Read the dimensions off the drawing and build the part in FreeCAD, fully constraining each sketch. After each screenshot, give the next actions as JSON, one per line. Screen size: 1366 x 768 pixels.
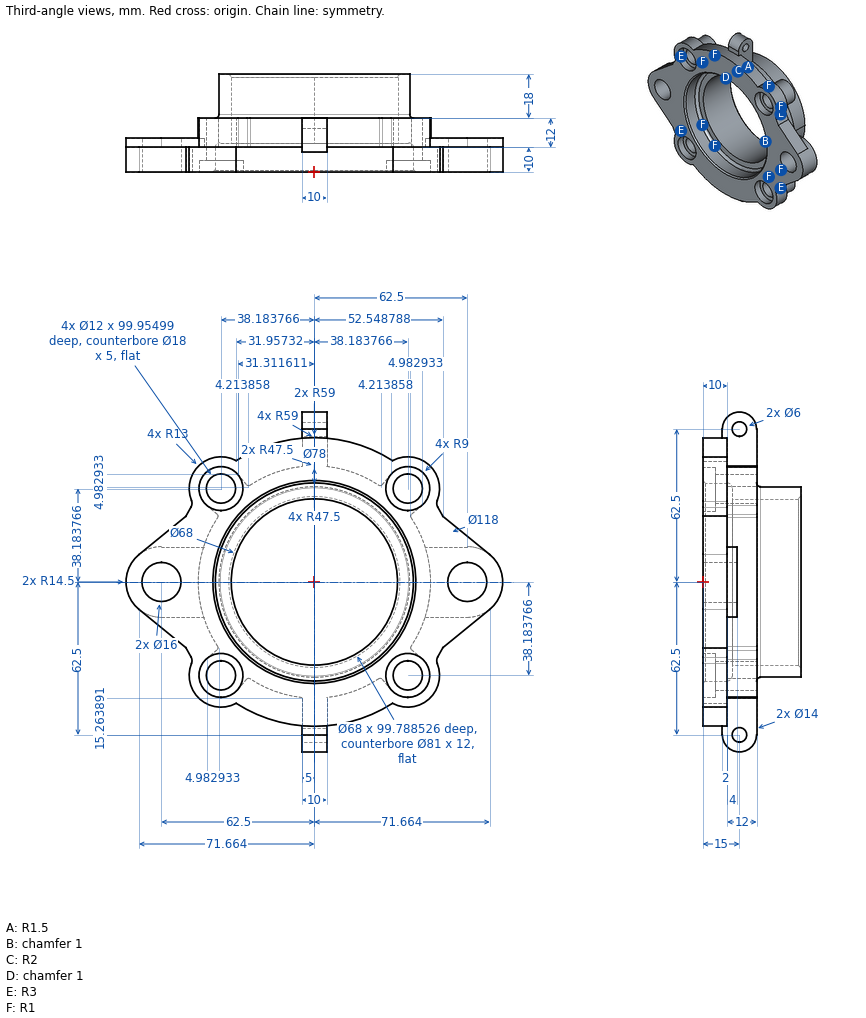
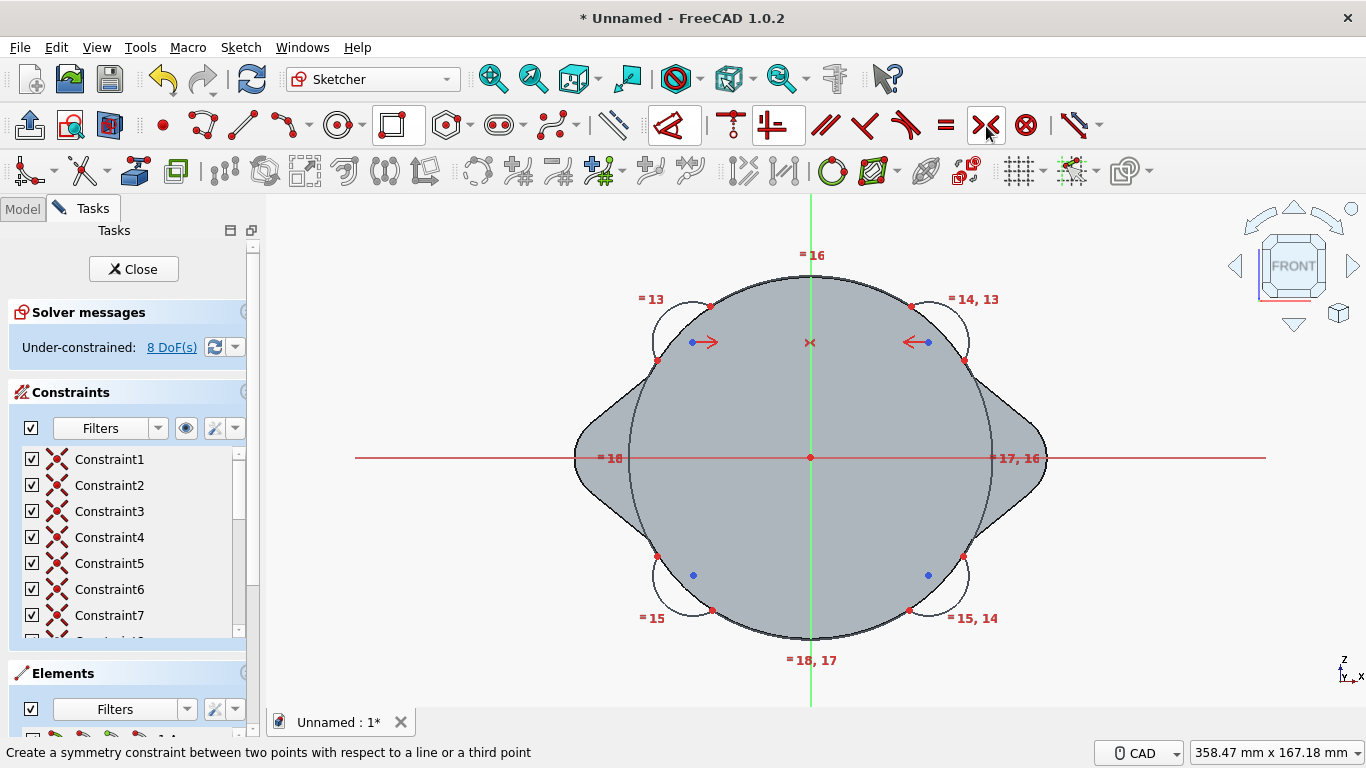
{"action": "left_click", "coordinate": [929, 342]}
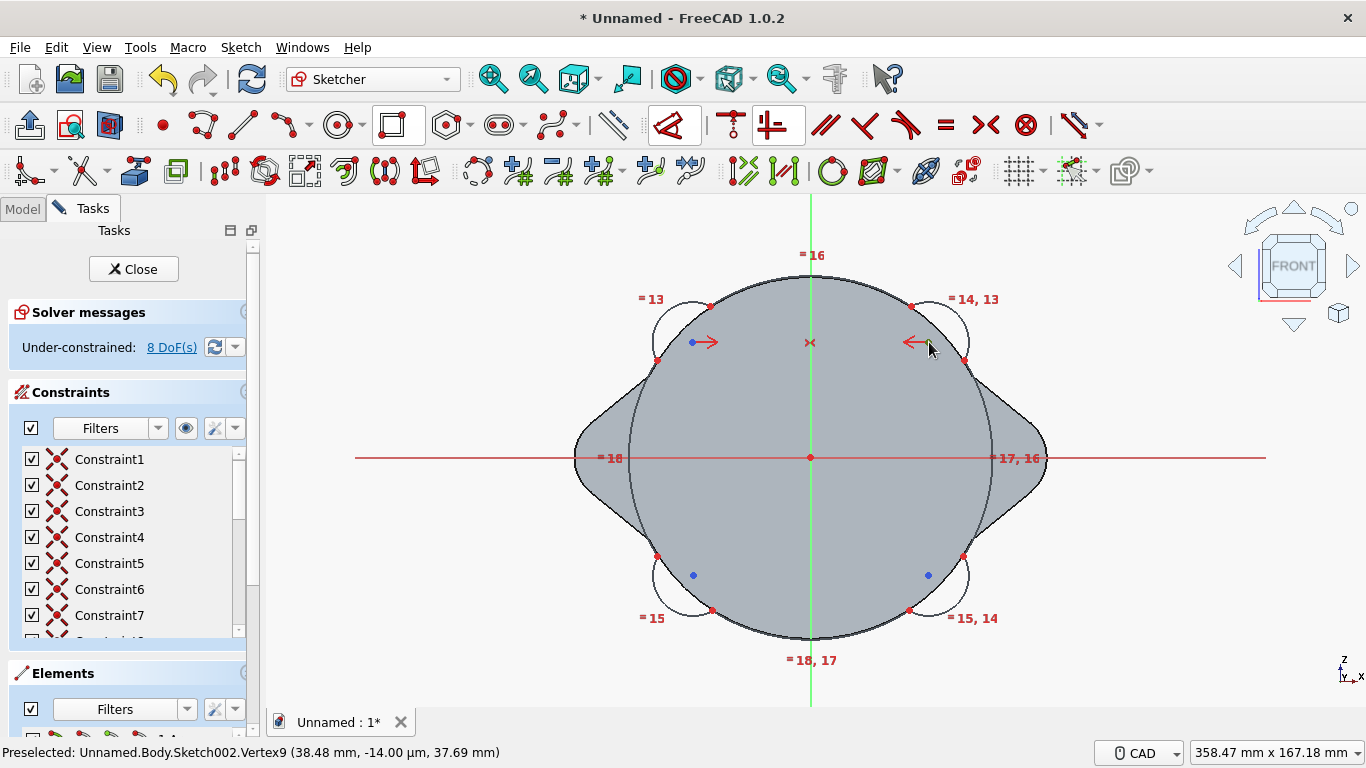
{"action": "left_click", "coordinate": [929, 576]}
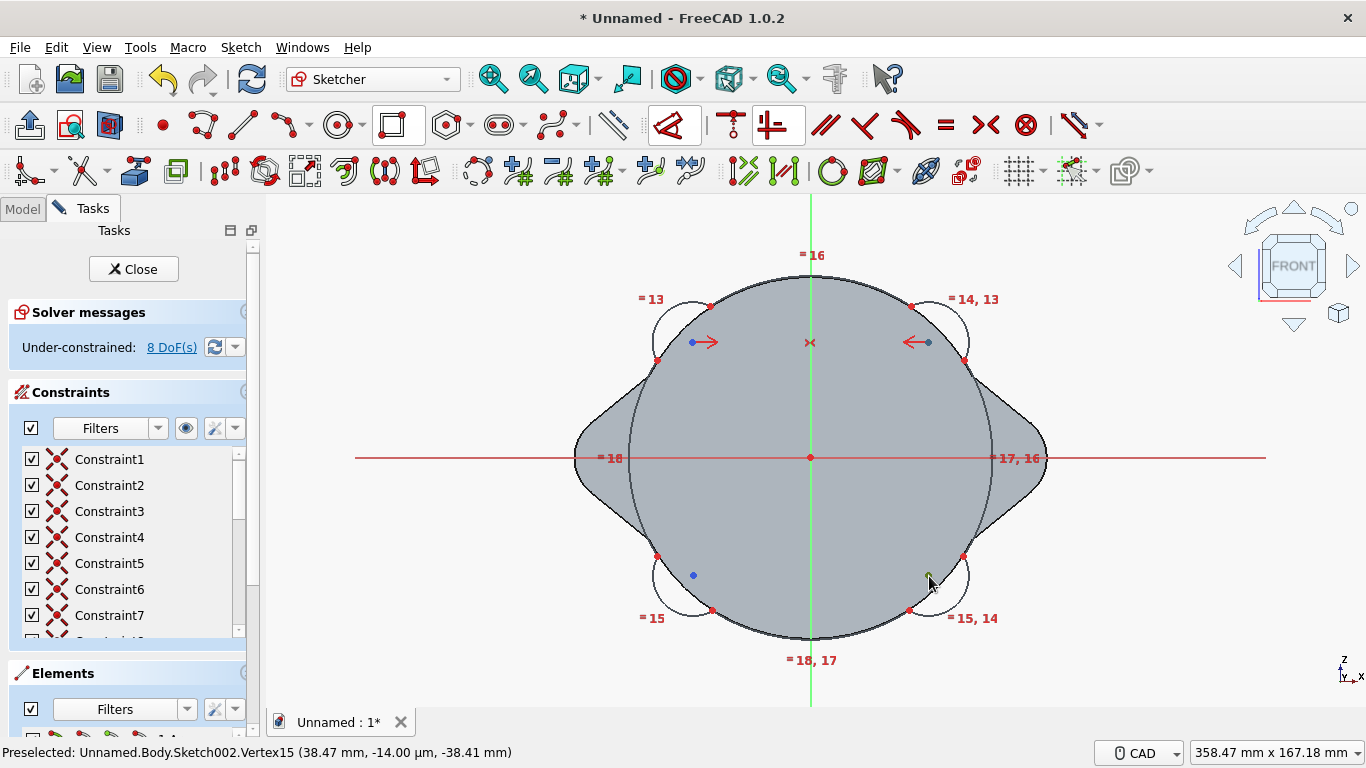
{"action": "left_click", "coordinate": [359, 458]}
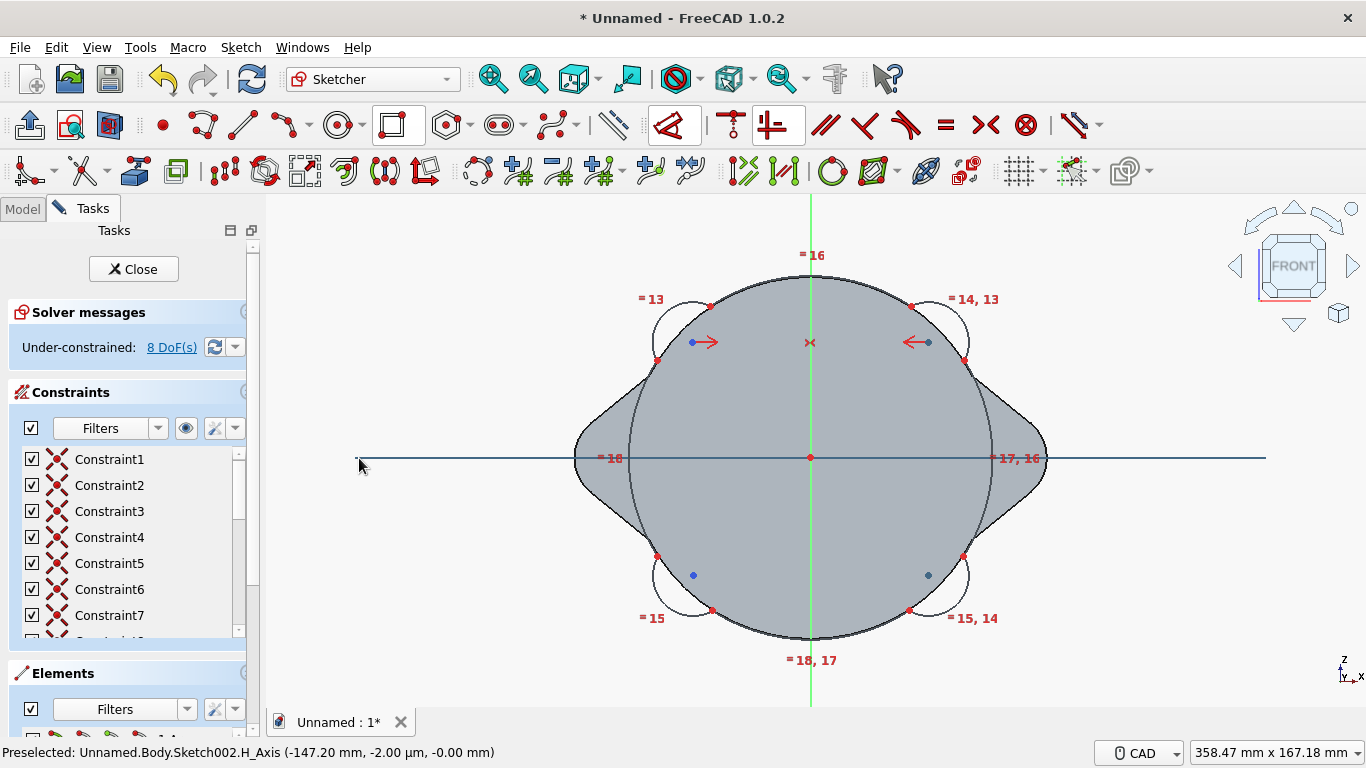
{"action": "left_click", "coordinate": [986, 126]}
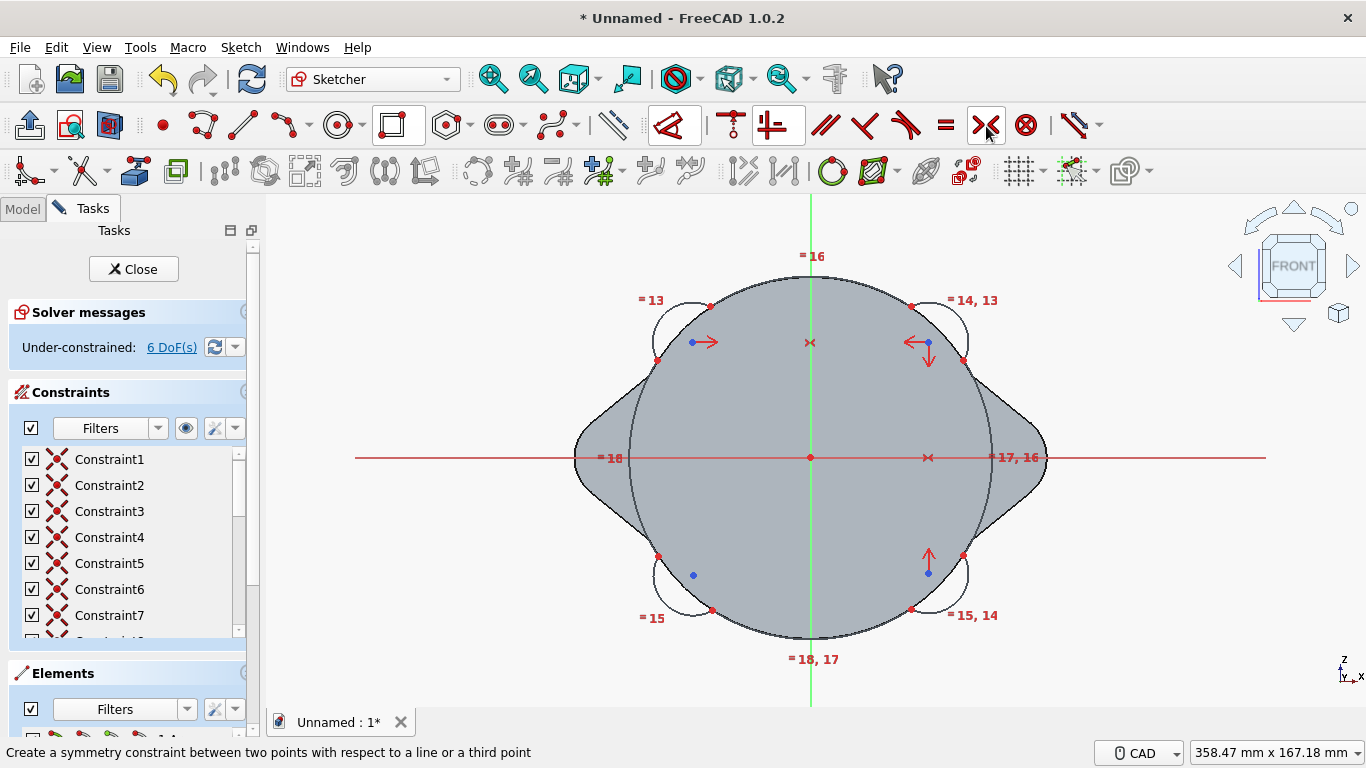
{"action": "left_click", "coordinate": [693, 342]}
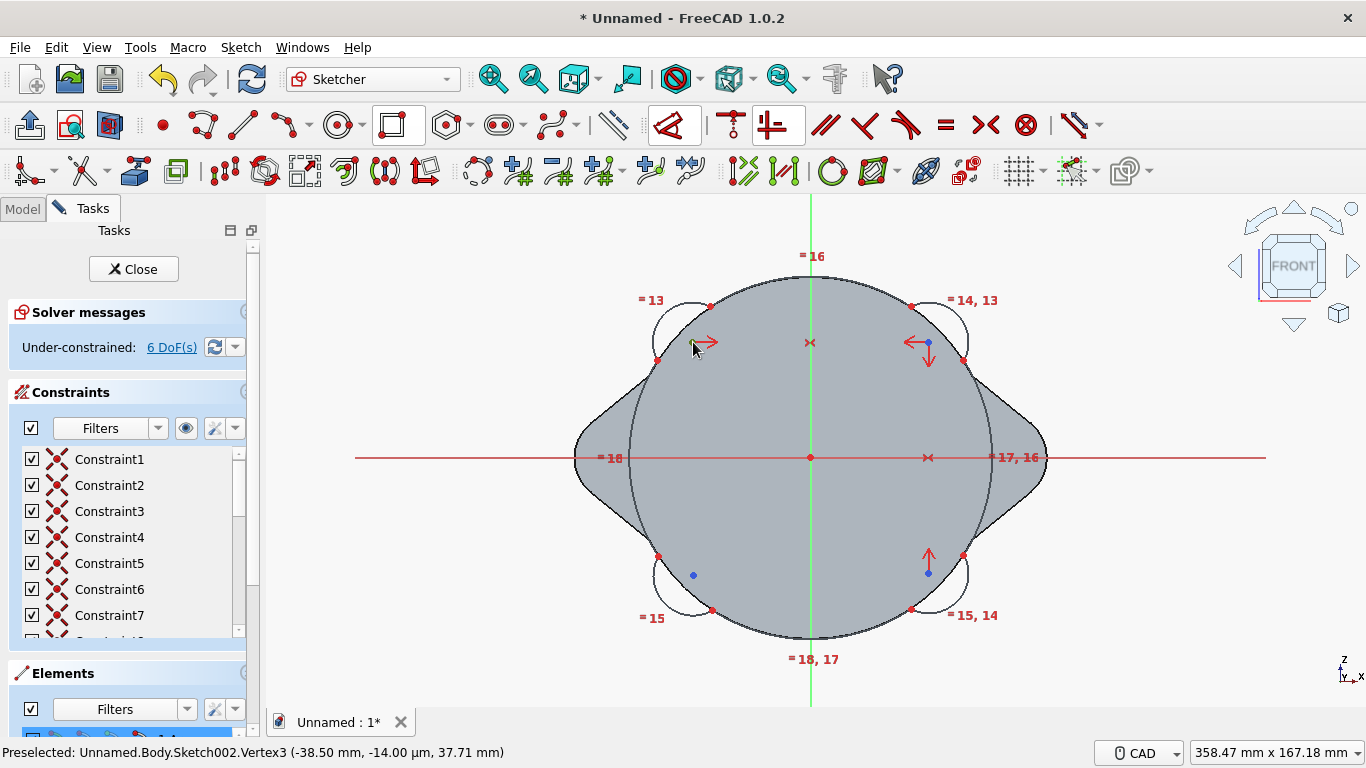
{"action": "left_click", "coordinate": [693, 576]}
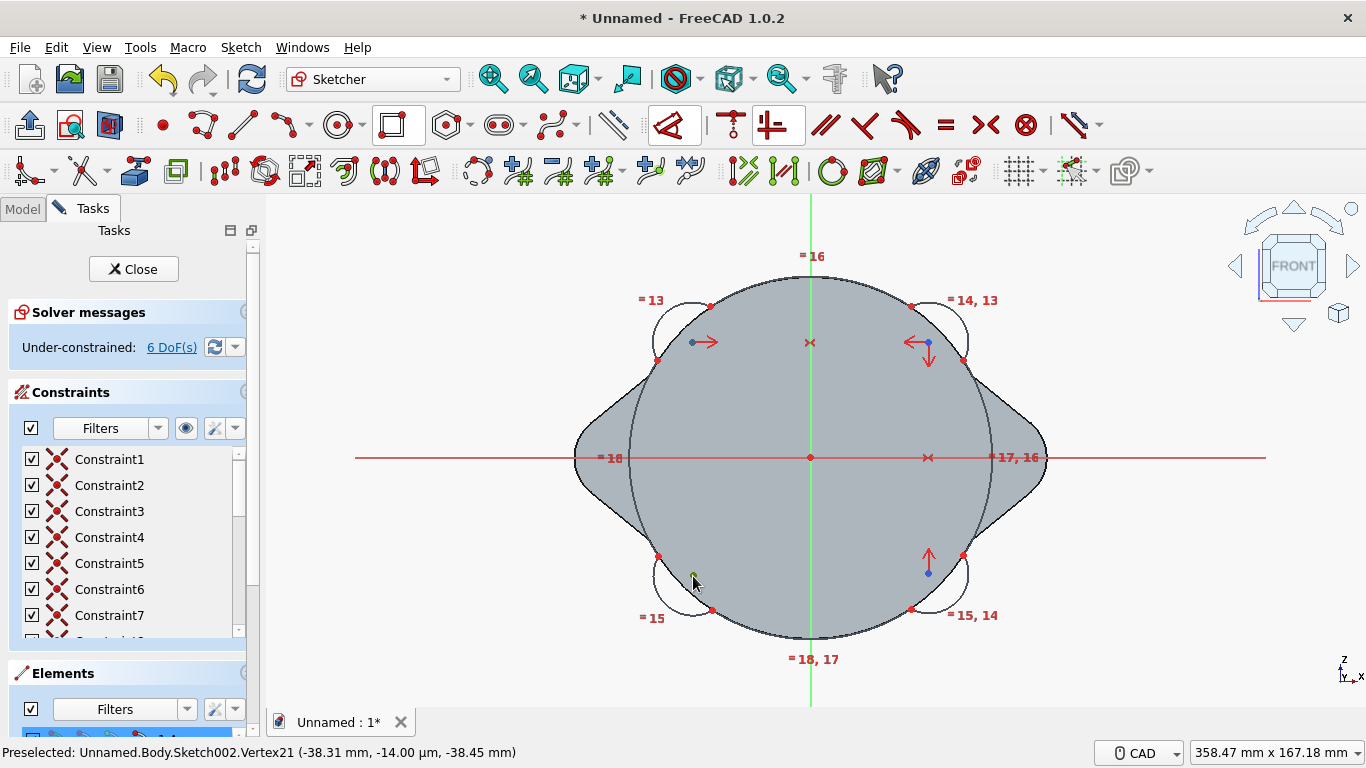
{"action": "left_click", "coordinate": [359, 458]}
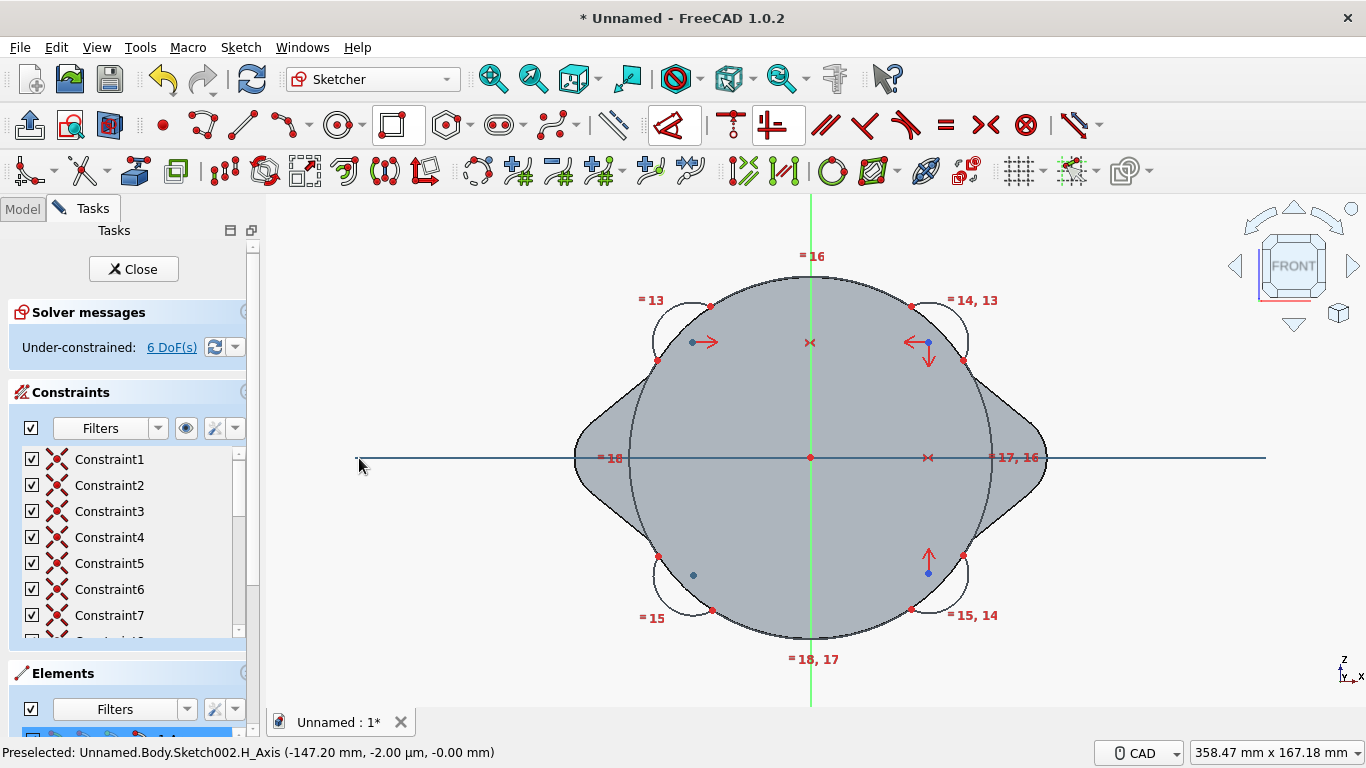
{"action": "left_click", "coordinate": [986, 126]}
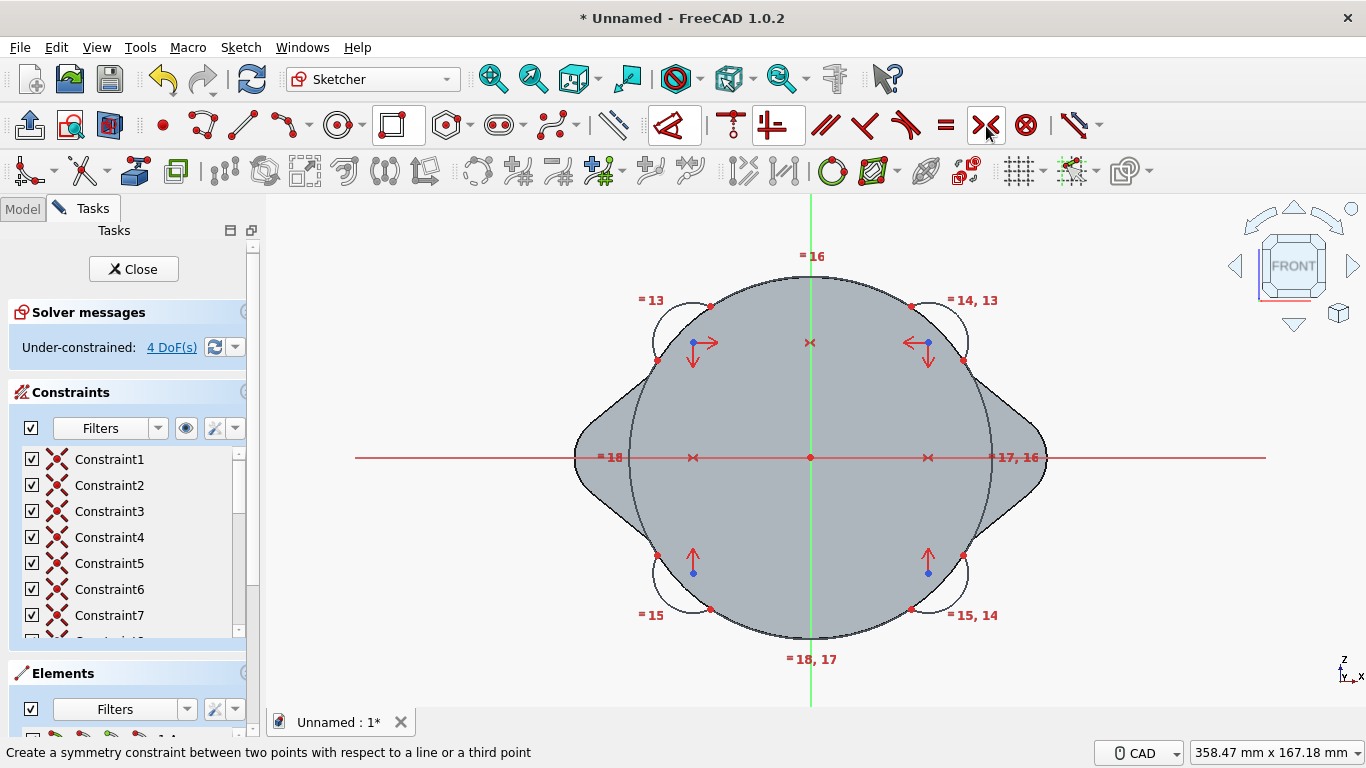
{"action": "left_click", "coordinate": [681, 305]}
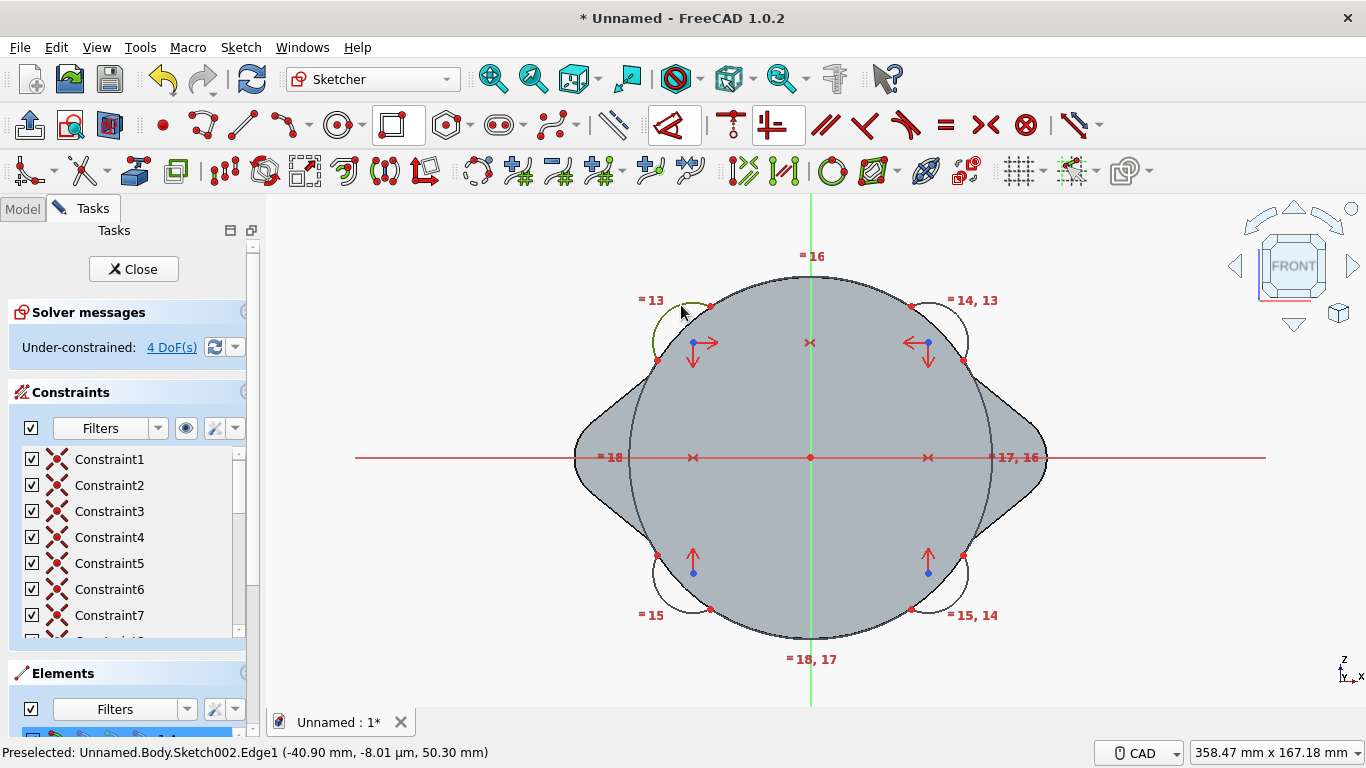
{"action": "left_click", "coordinate": [696, 126]}